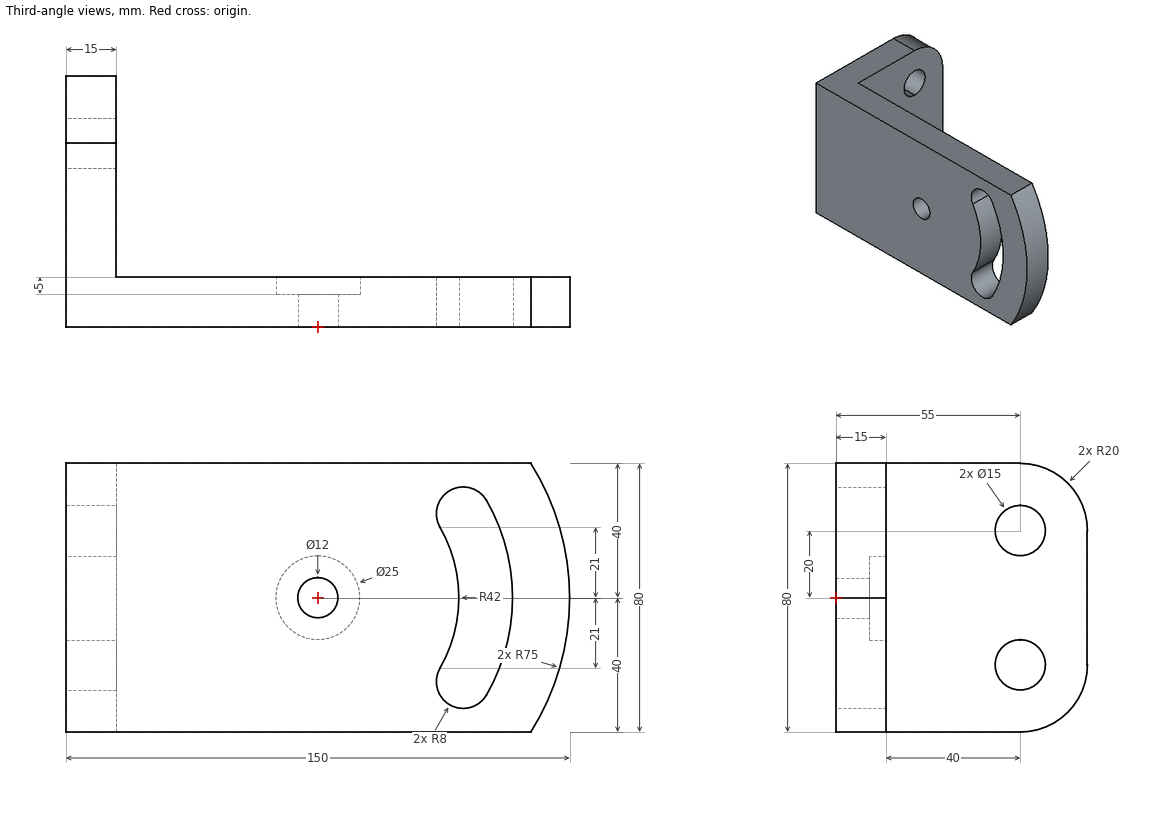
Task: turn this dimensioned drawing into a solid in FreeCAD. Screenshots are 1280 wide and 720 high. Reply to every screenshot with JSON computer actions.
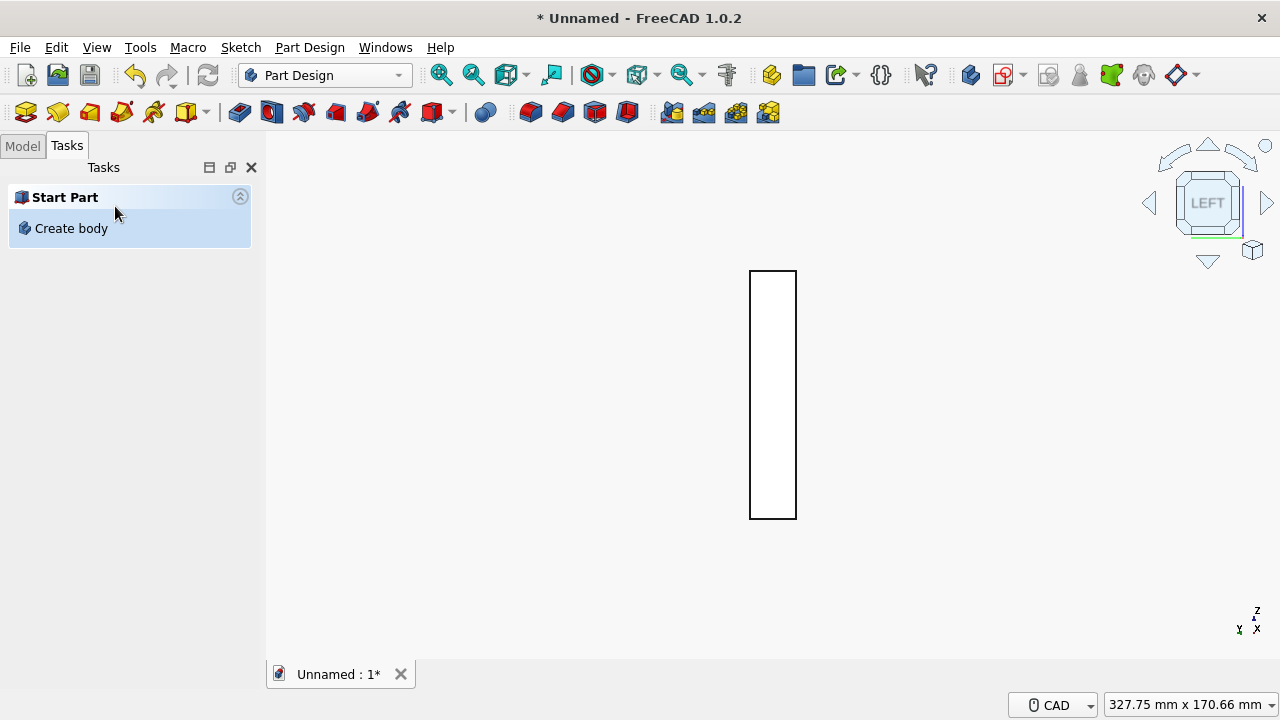
{"action": "left_click", "coordinate": [773, 394]}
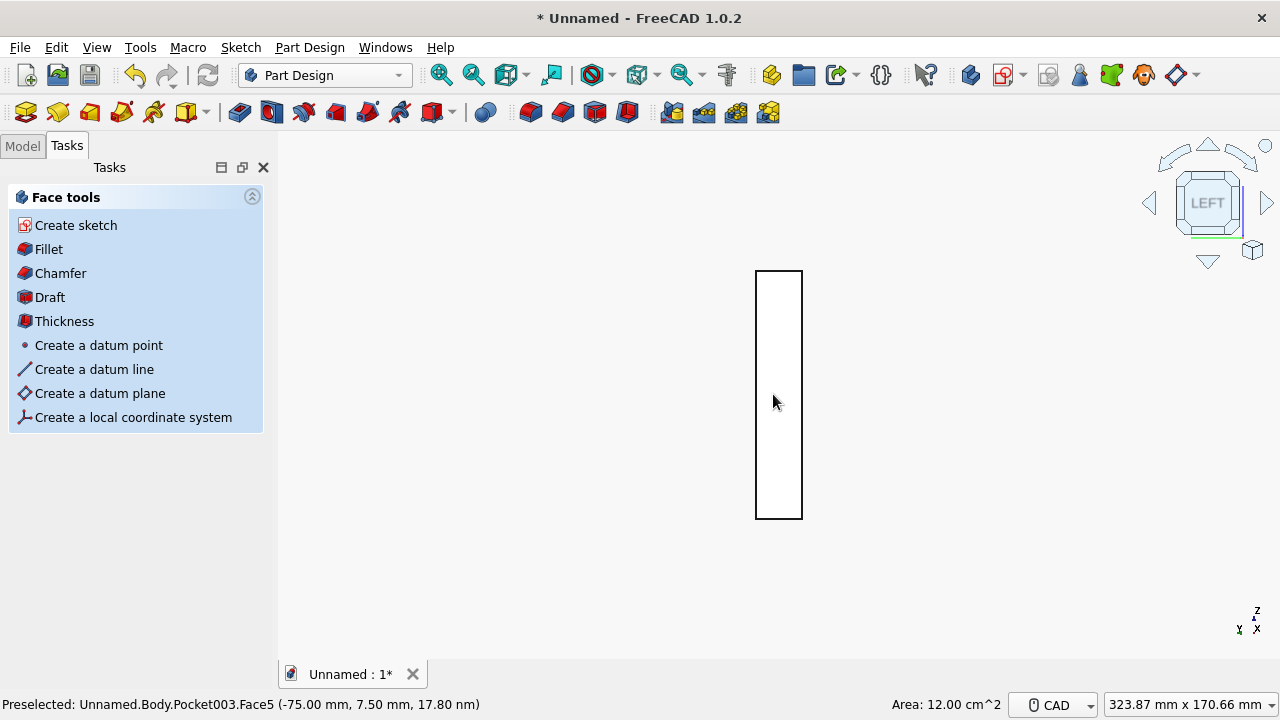
{"action": "left_click", "coordinate": [1004, 76]}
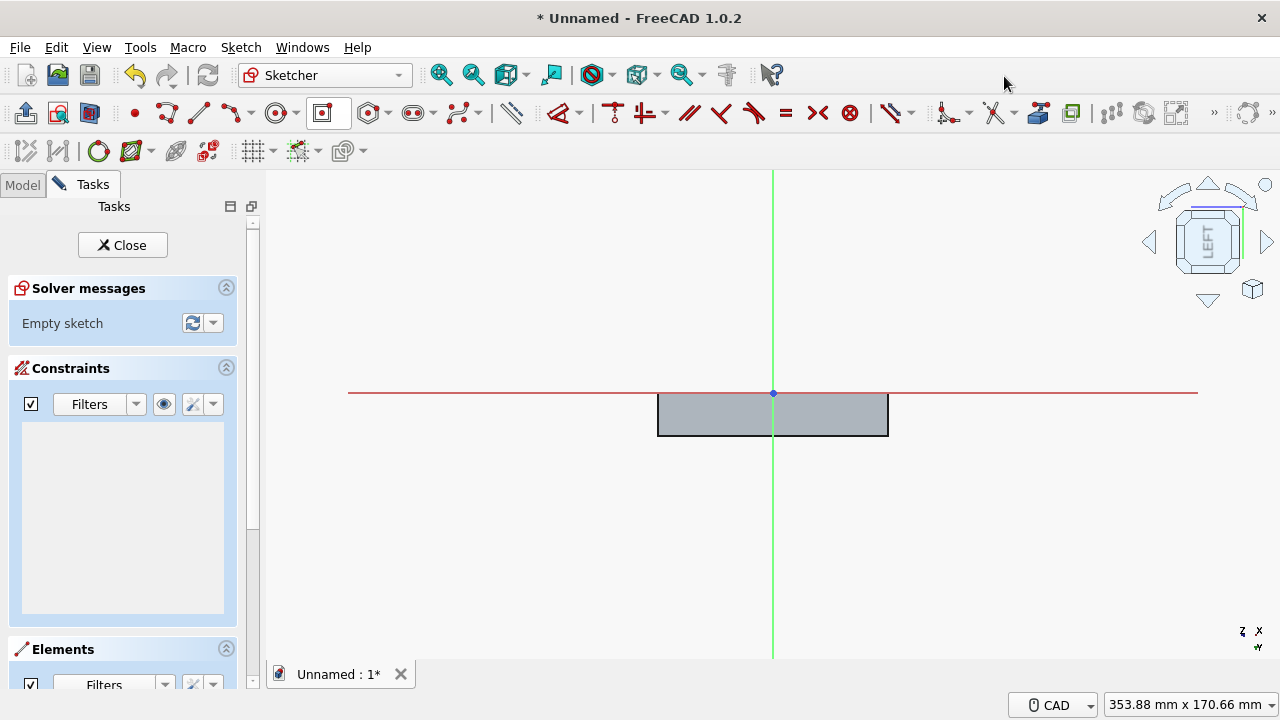
{"action": "scroll", "coordinate": [912, 631], "scroll_direction": "up", "scroll_amount": 2}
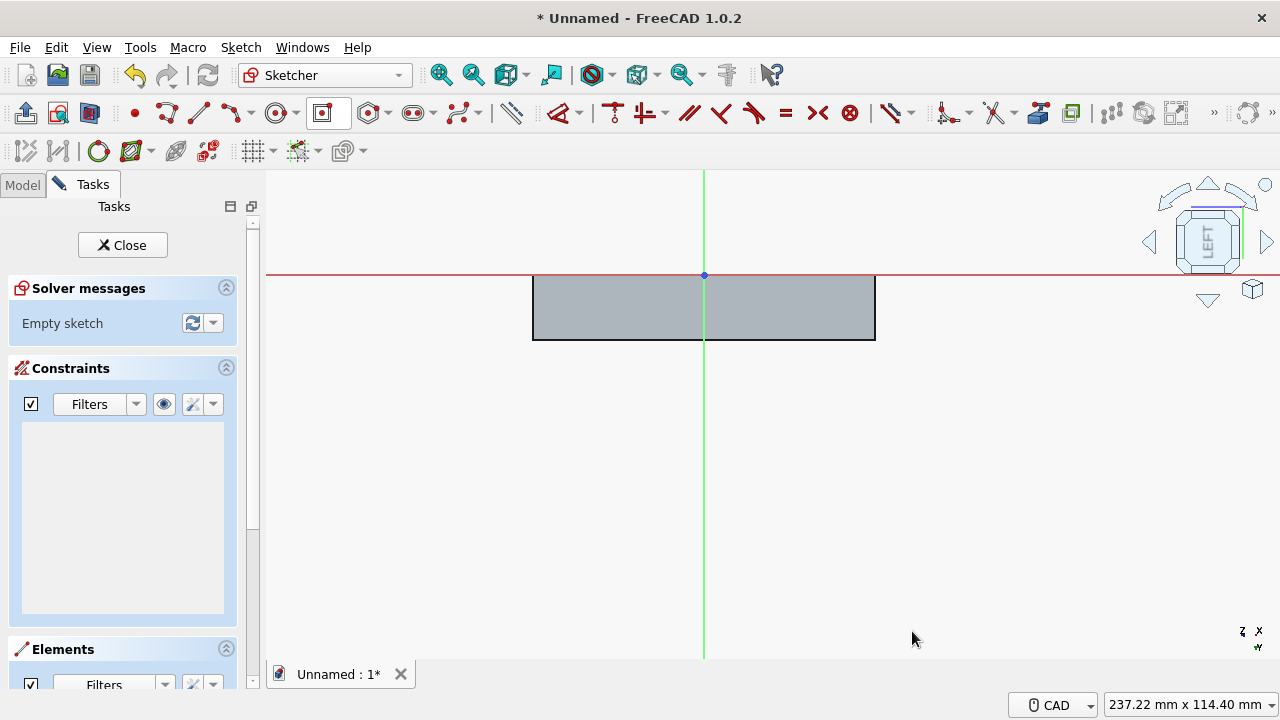
{"action": "left_click", "coordinate": [168, 114]}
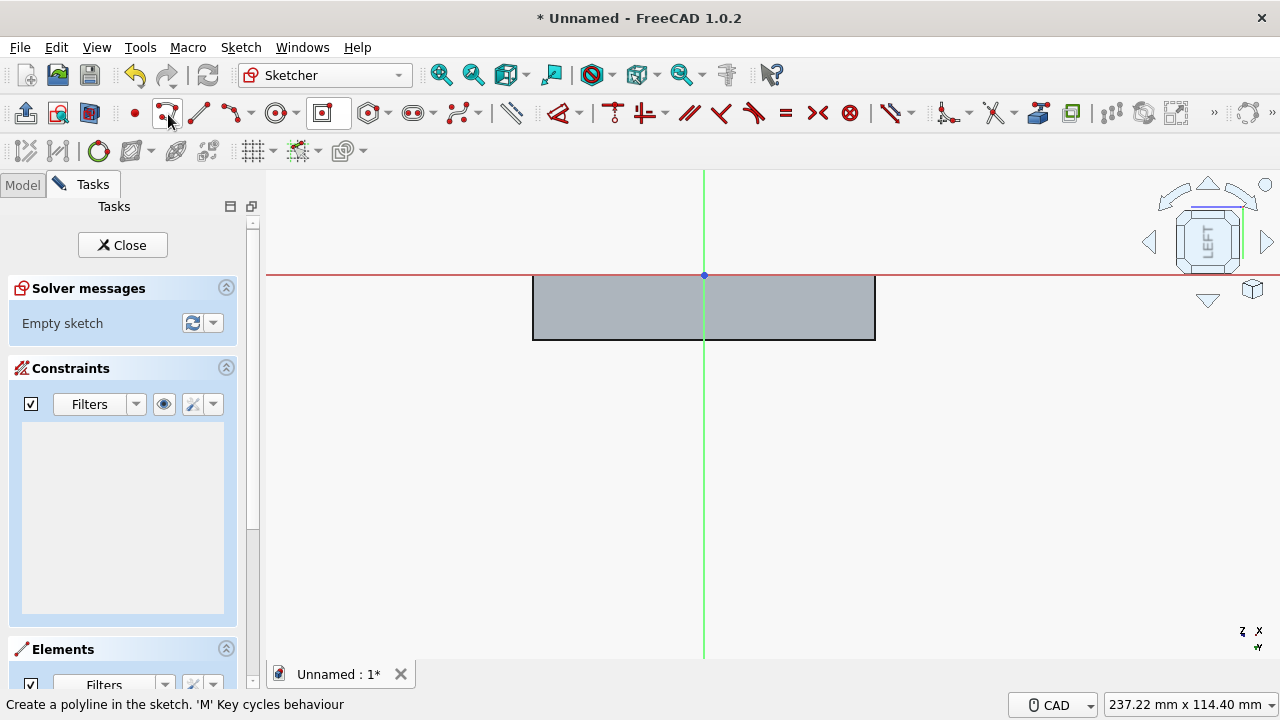
{"action": "left_click", "coordinate": [875, 511]}
{"action": "left_click", "coordinate": [875, 340]}
{"action": "left_click", "coordinate": [533, 340]}
{"action": "left_click", "coordinate": [533, 511]}
{"action": "right_click", "coordinate": [533, 511]}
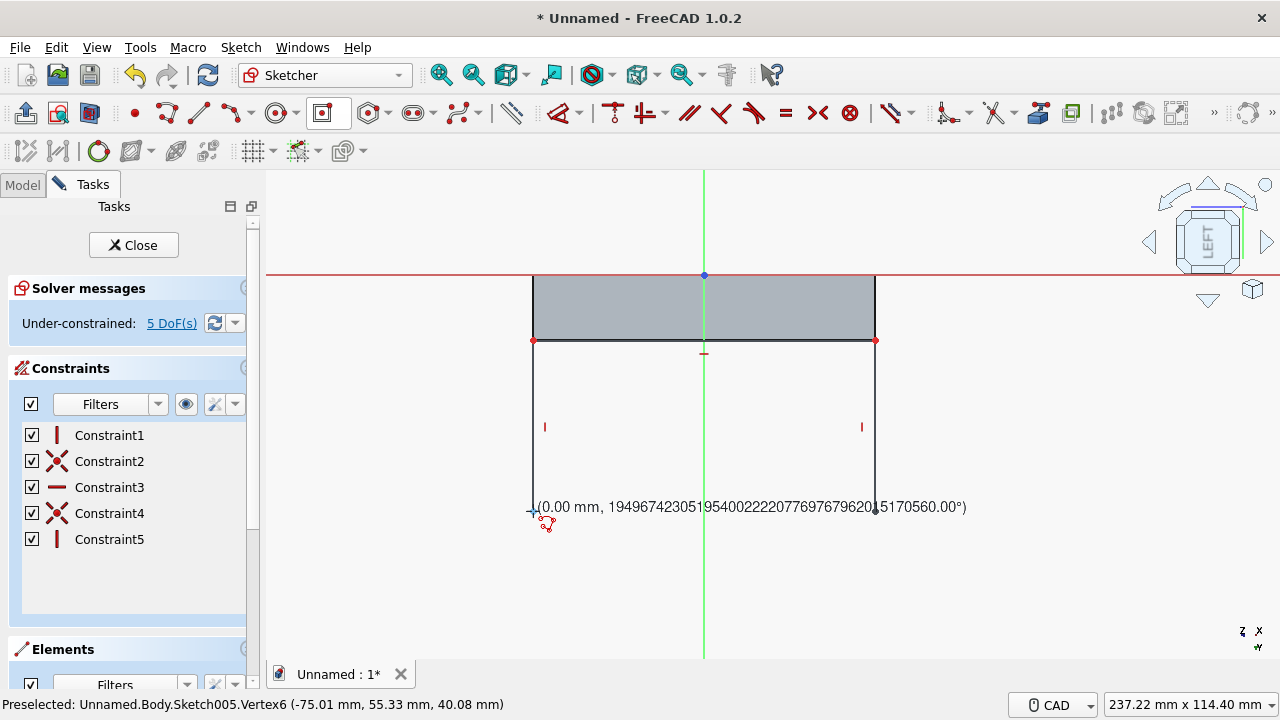
{"action": "left_click", "coordinate": [200, 114]}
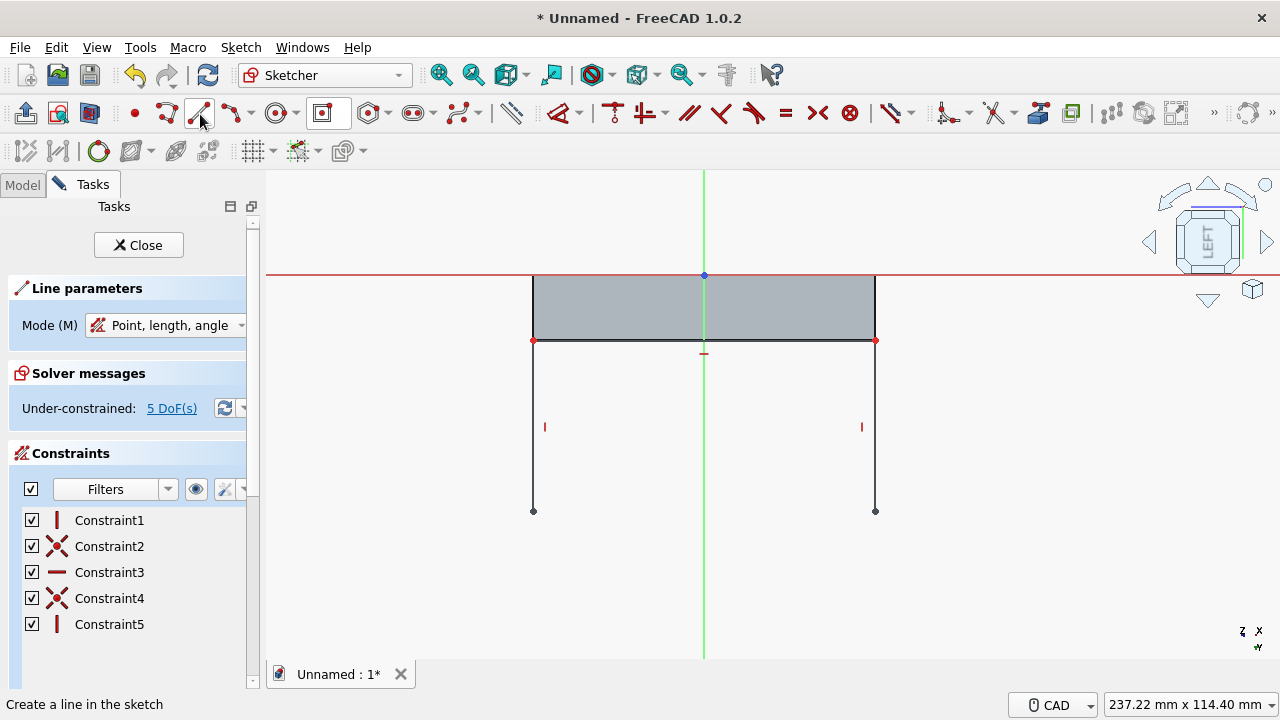
{"action": "left_click", "coordinate": [619, 596]}
{"action": "left_click", "coordinate": [790, 596]}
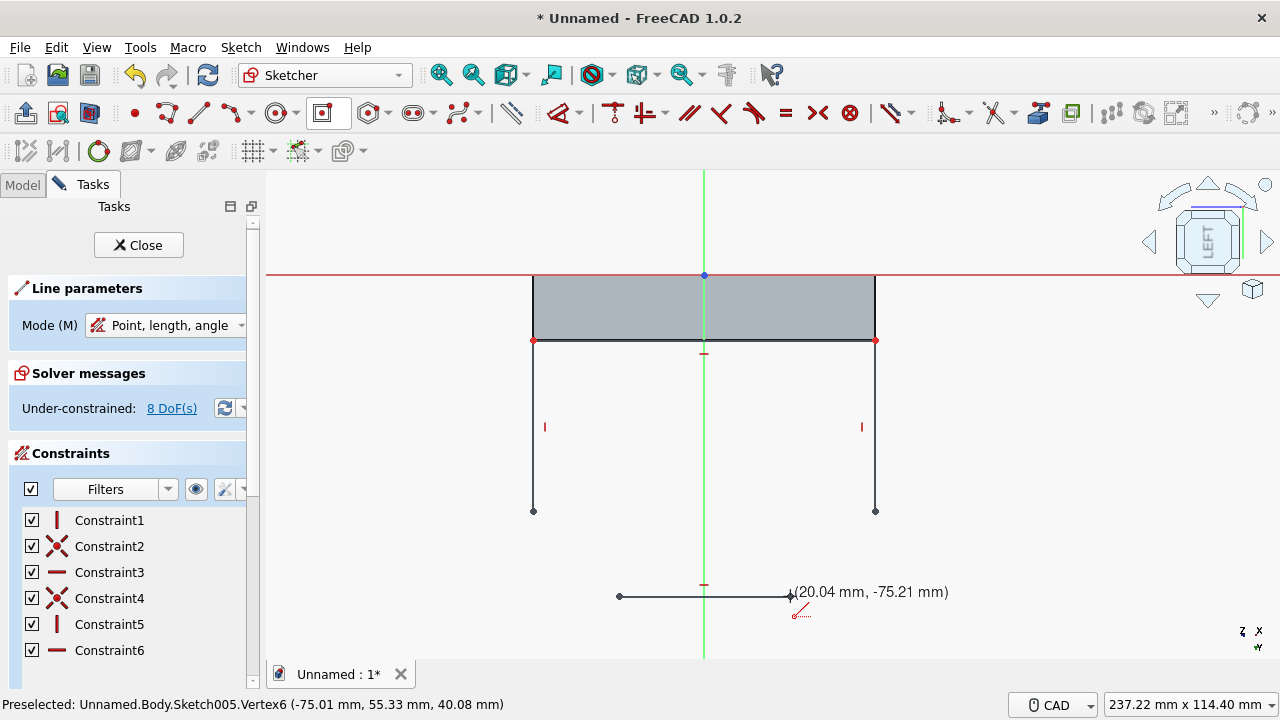
{"action": "left_click", "coordinate": [232, 114]}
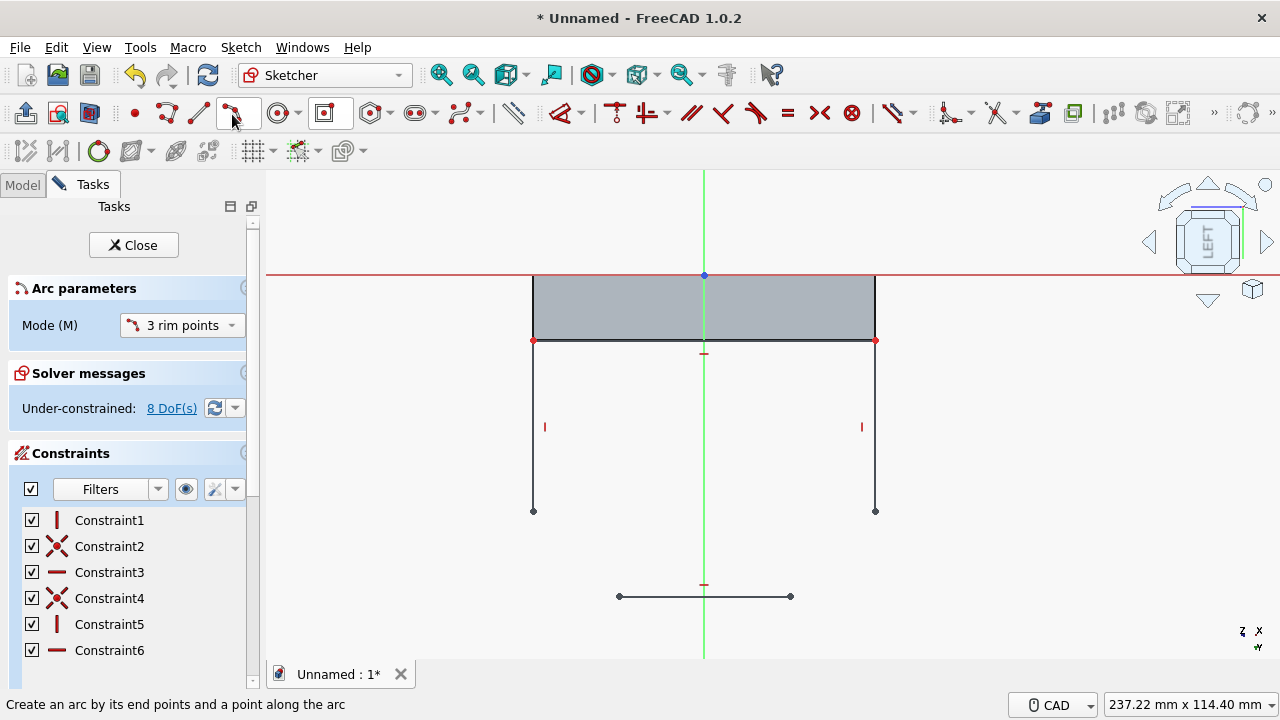
{"action": "left_click", "coordinate": [533, 512]}
{"action": "left_click", "coordinate": [619, 597]}
{"action": "left_click", "coordinate": [558, 571]}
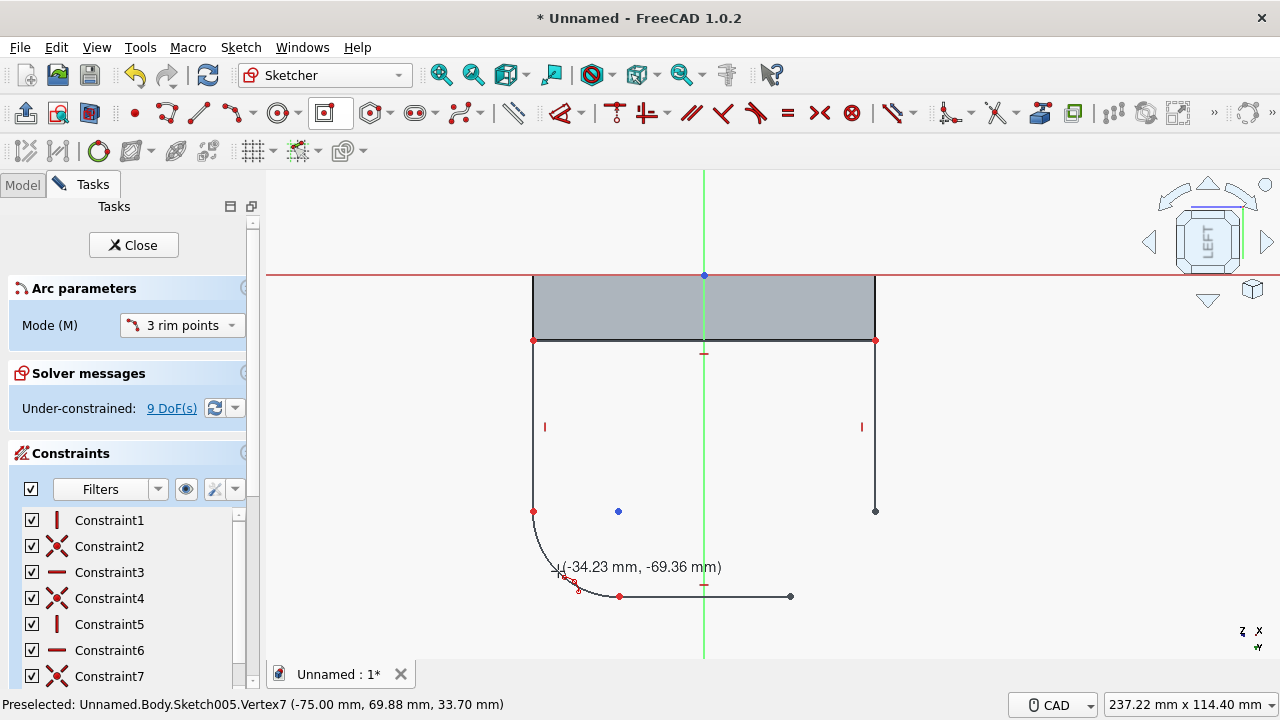
{"action": "left_click", "coordinate": [790, 597]}
{"action": "left_click", "coordinate": [875, 512]}
{"action": "left_click", "coordinate": [850, 571]}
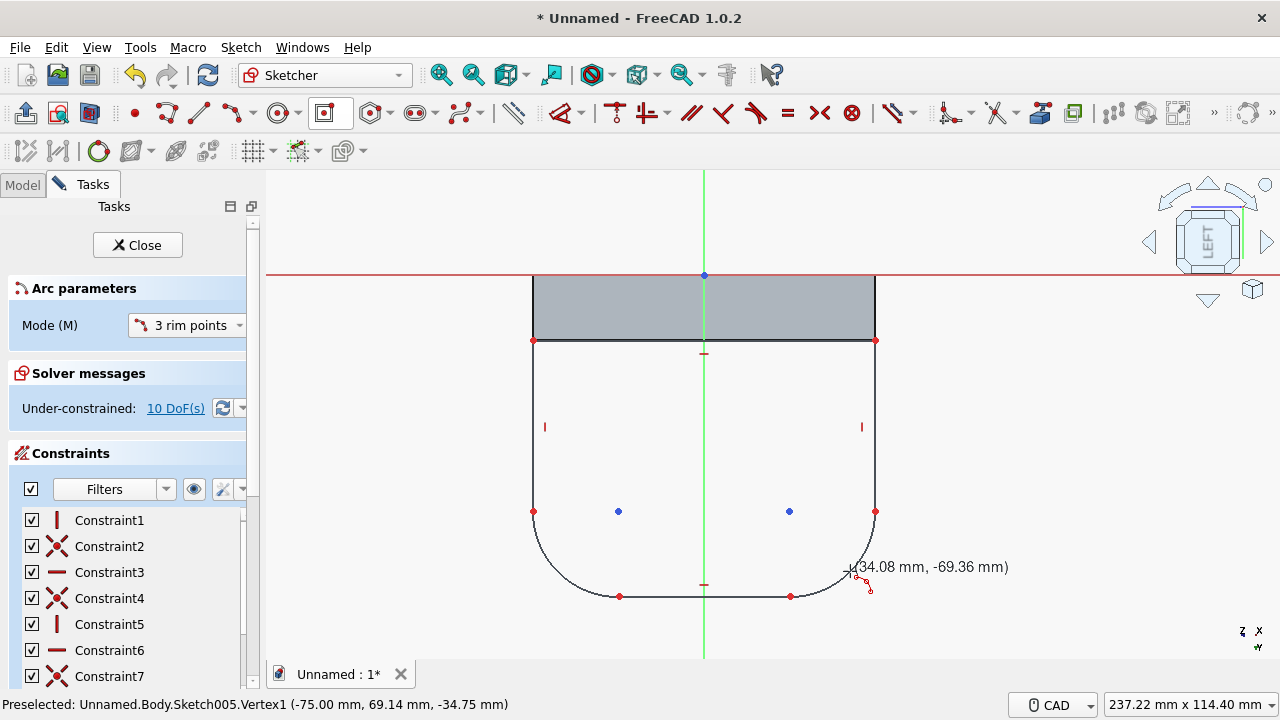
{"action": "left_click", "coordinate": [278, 114]}